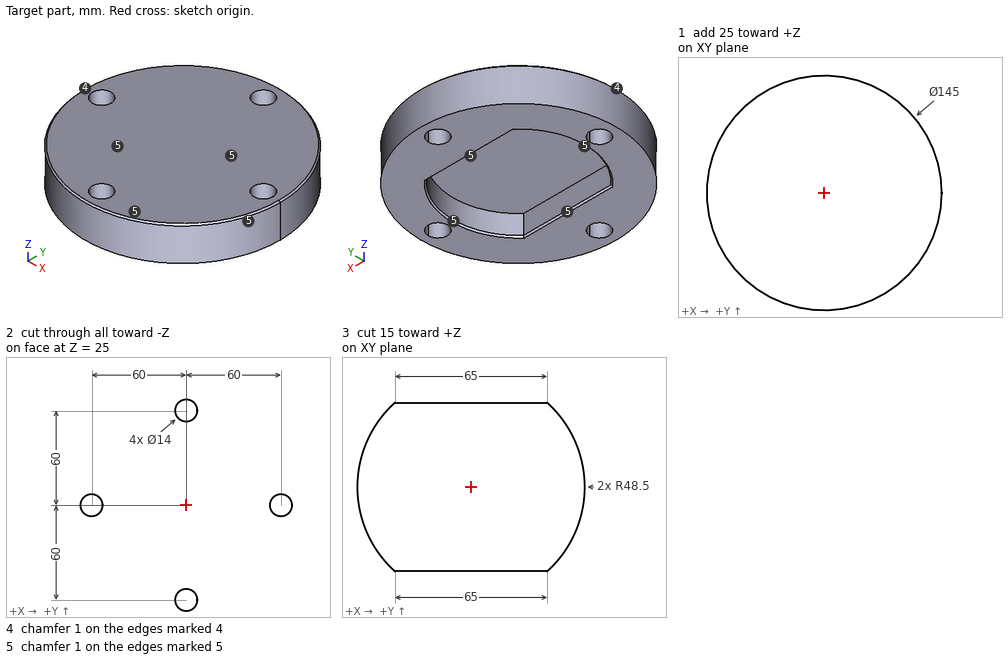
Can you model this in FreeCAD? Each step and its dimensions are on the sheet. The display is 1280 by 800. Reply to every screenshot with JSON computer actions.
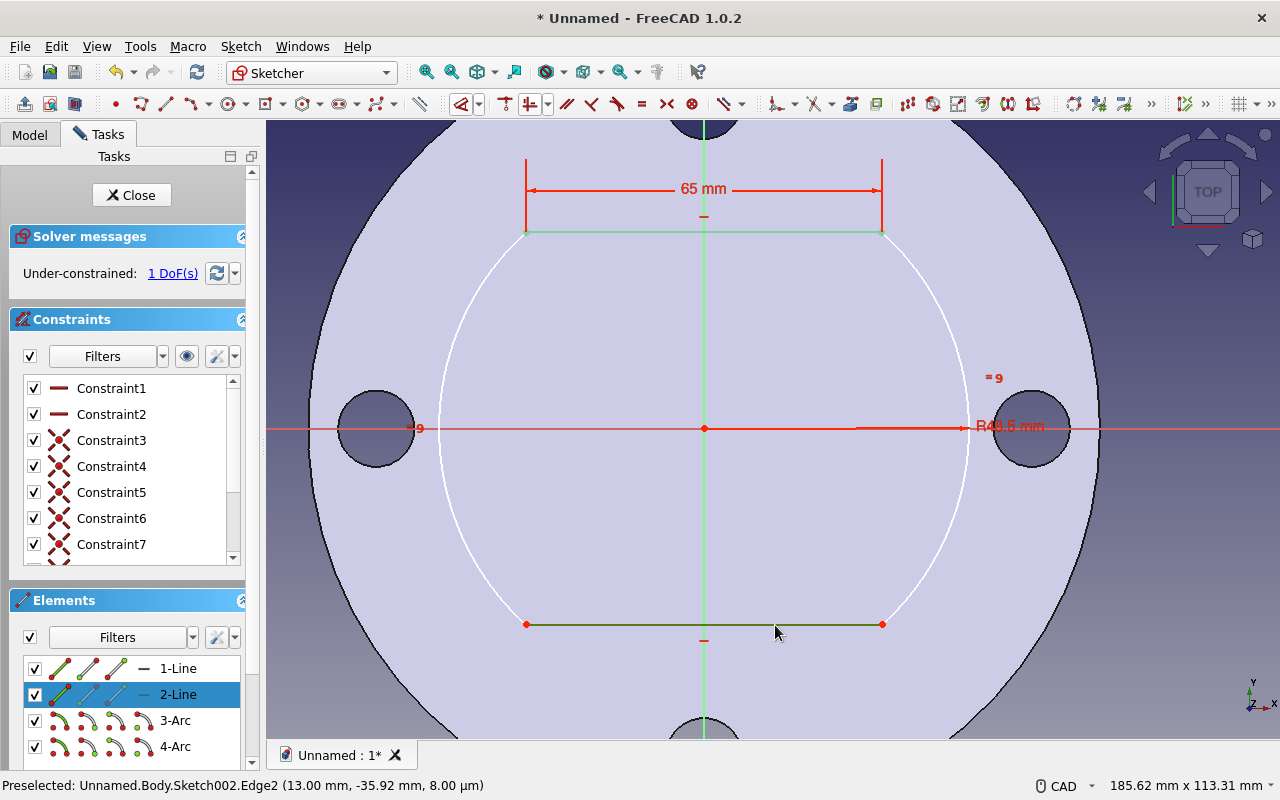
{"action": "left_click", "coordinate": [478, 104]}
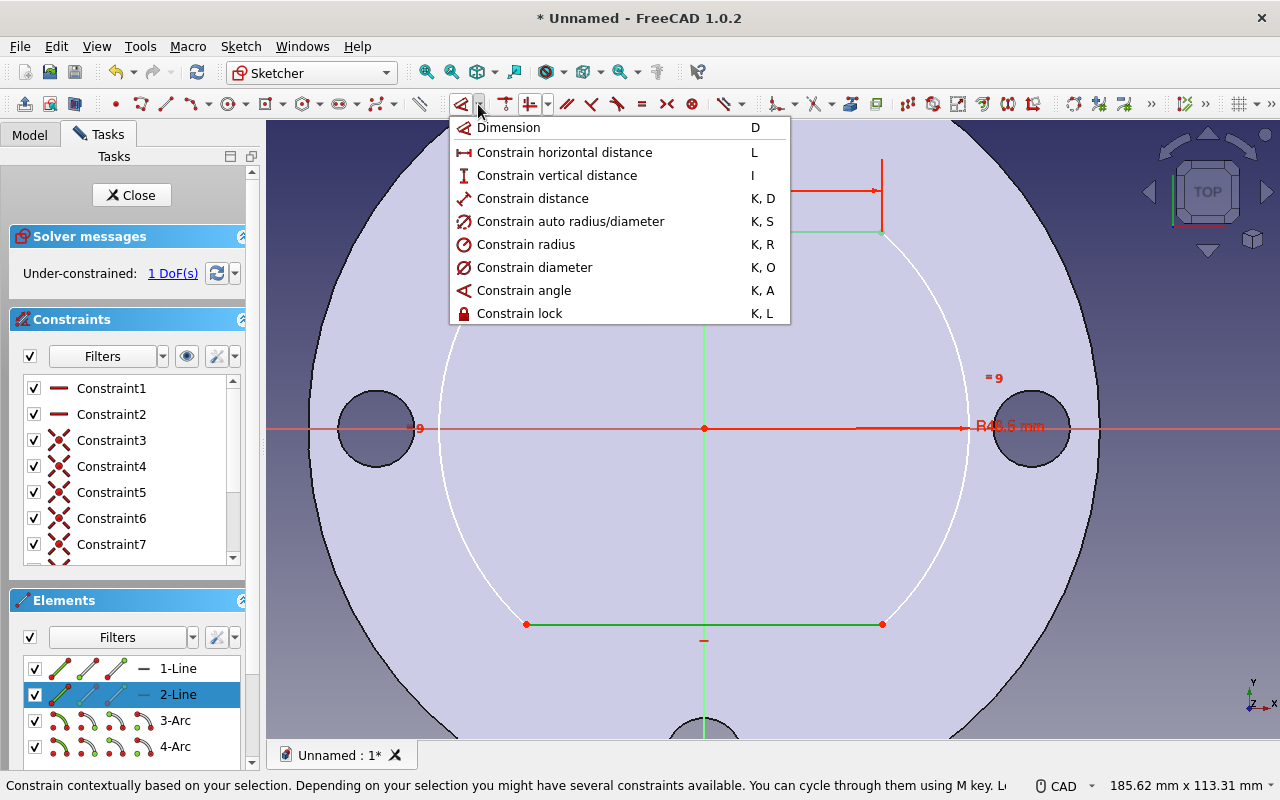
{"action": "left_click", "coordinate": [620, 152]}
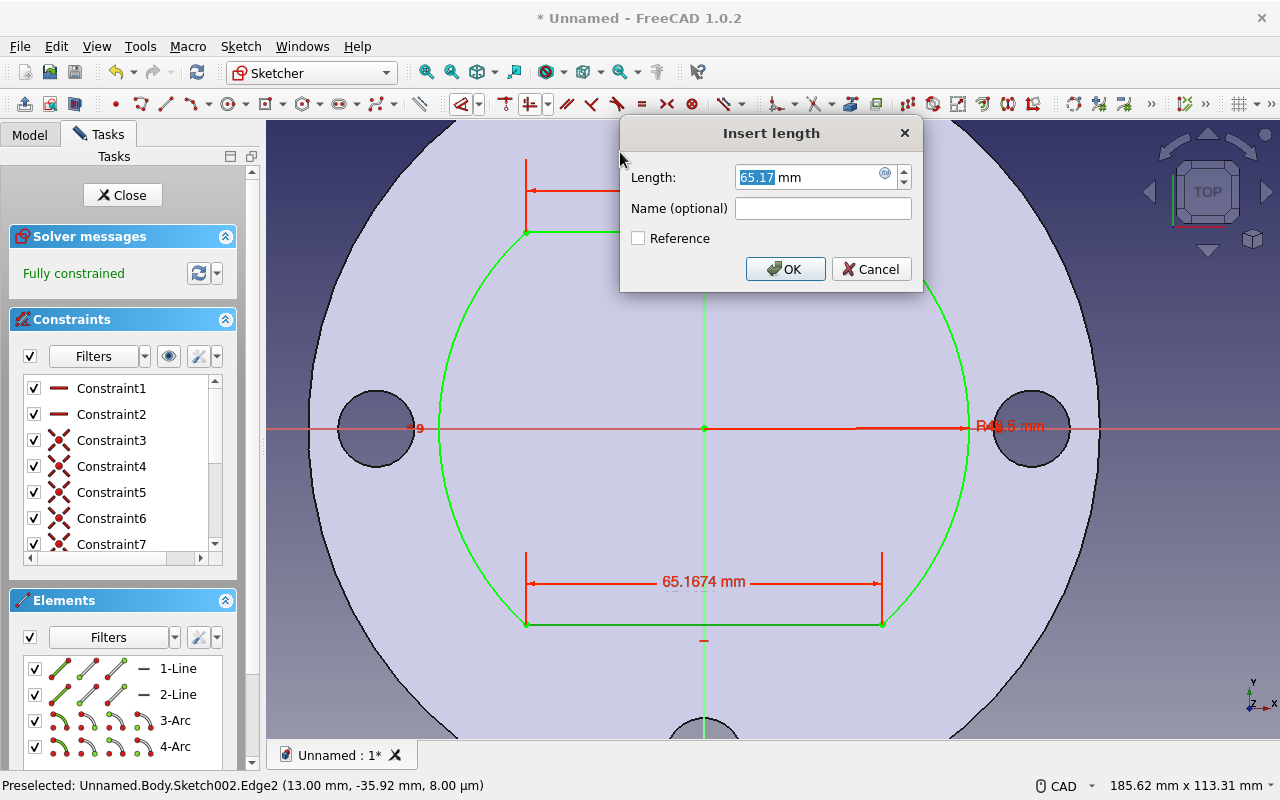
{"action": "type", "text": "65"}
{"action": "key", "text": "Return"}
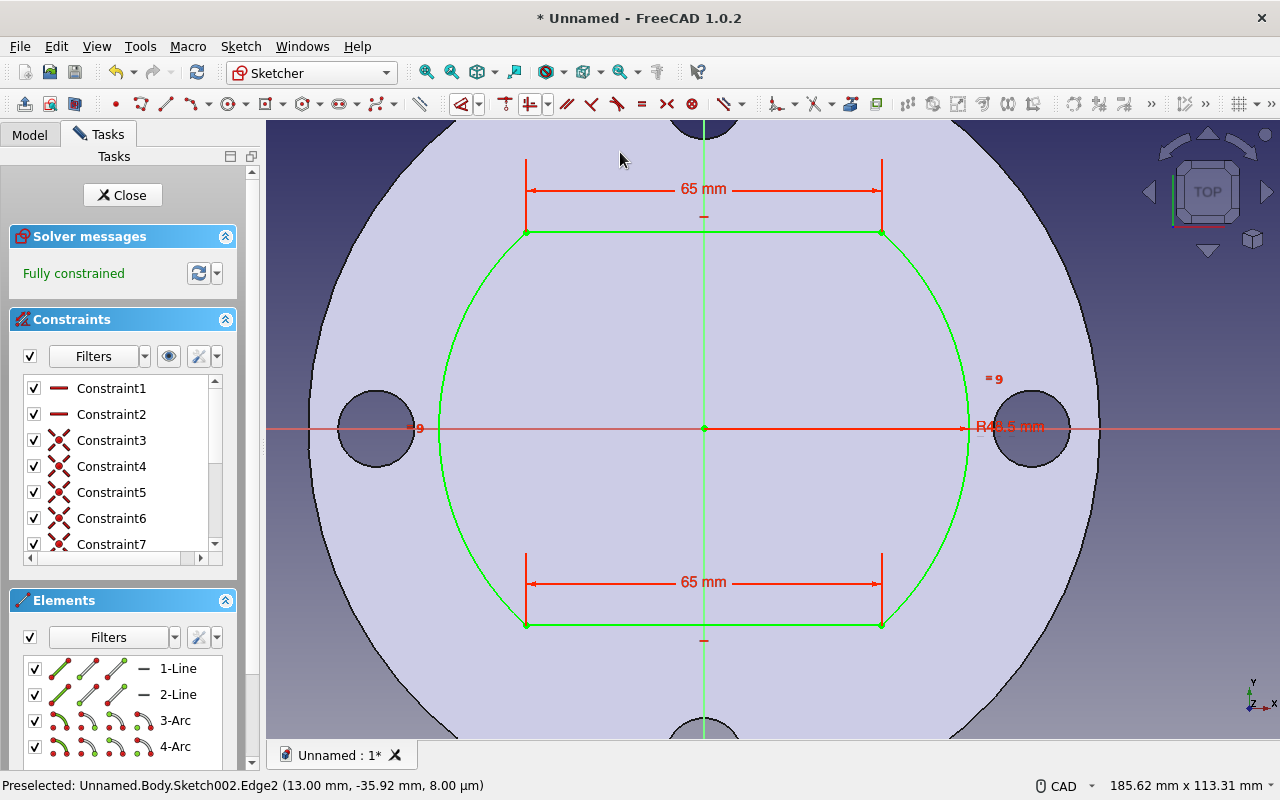
{"action": "left_click", "coordinate": [123, 195]}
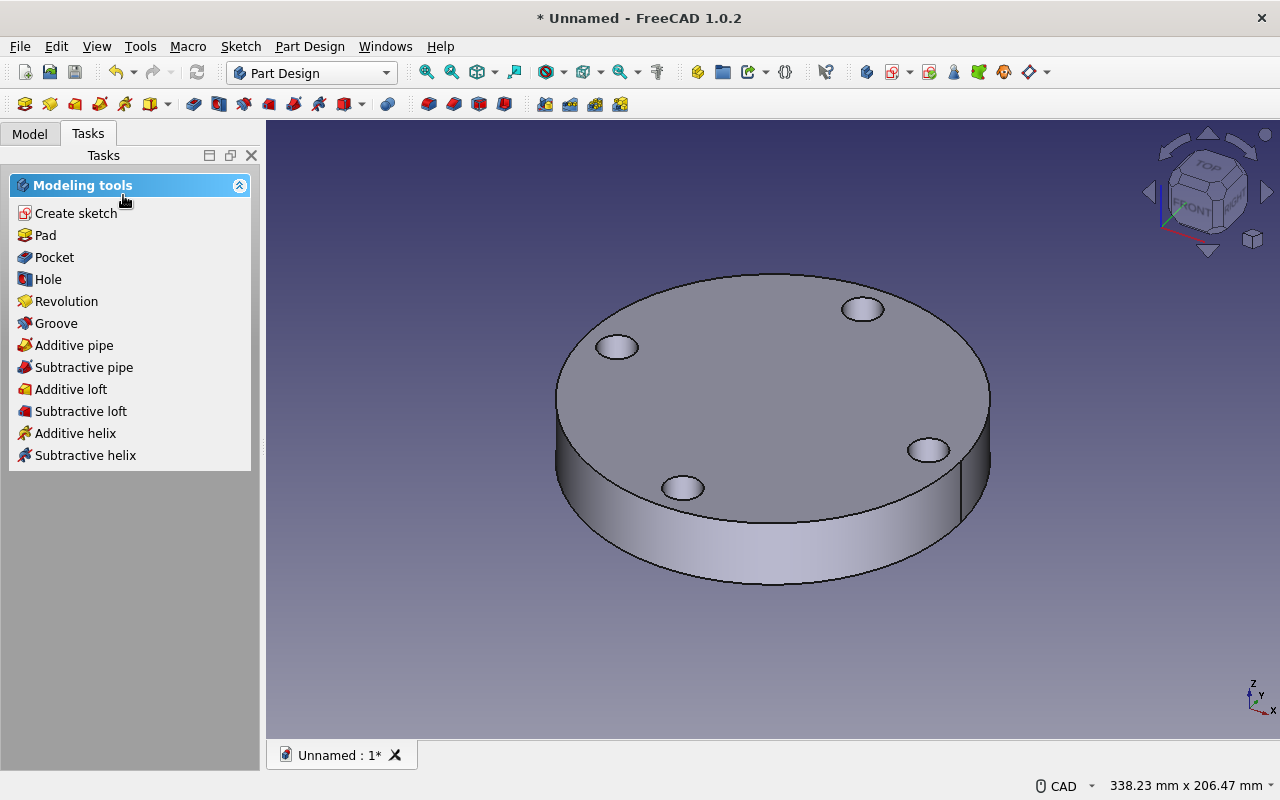
{"action": "left_click", "coordinate": [194, 104]}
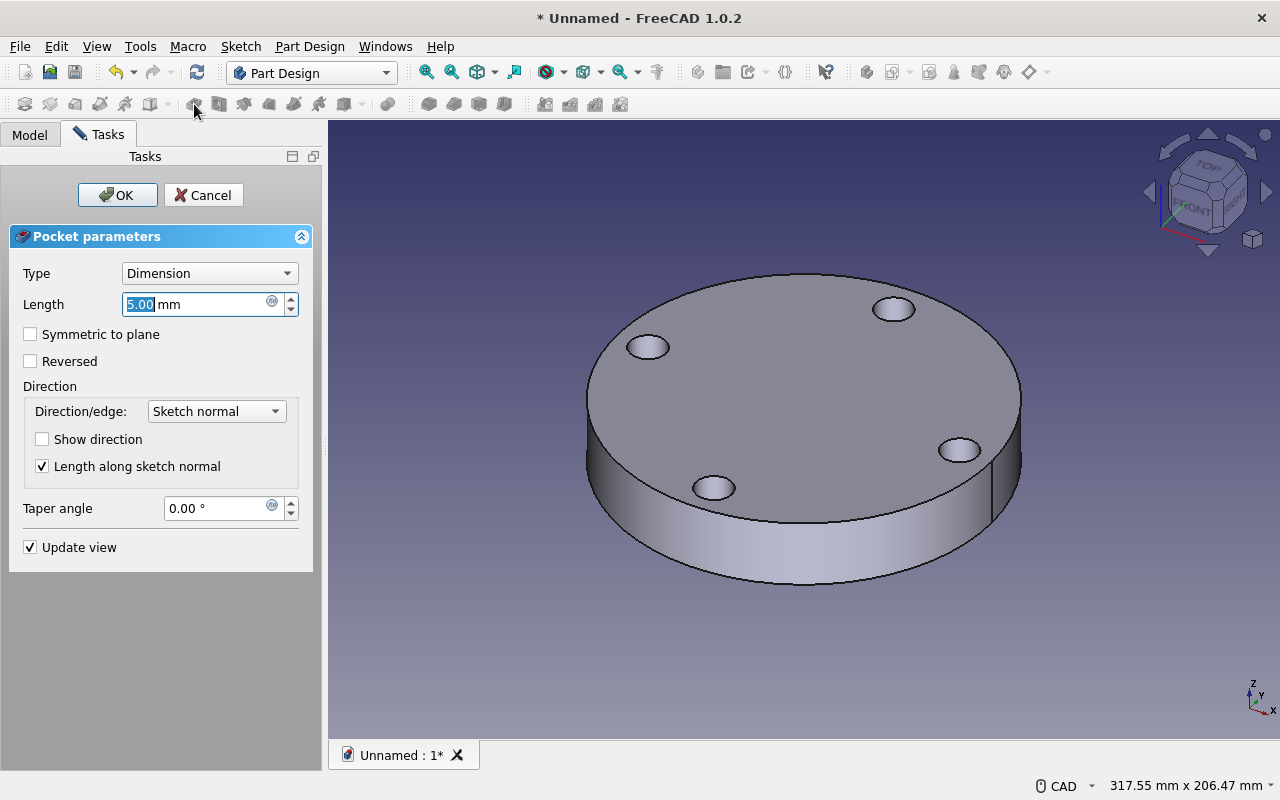
{"action": "type", "text": "15"}
{"action": "key", "text": "Tab"}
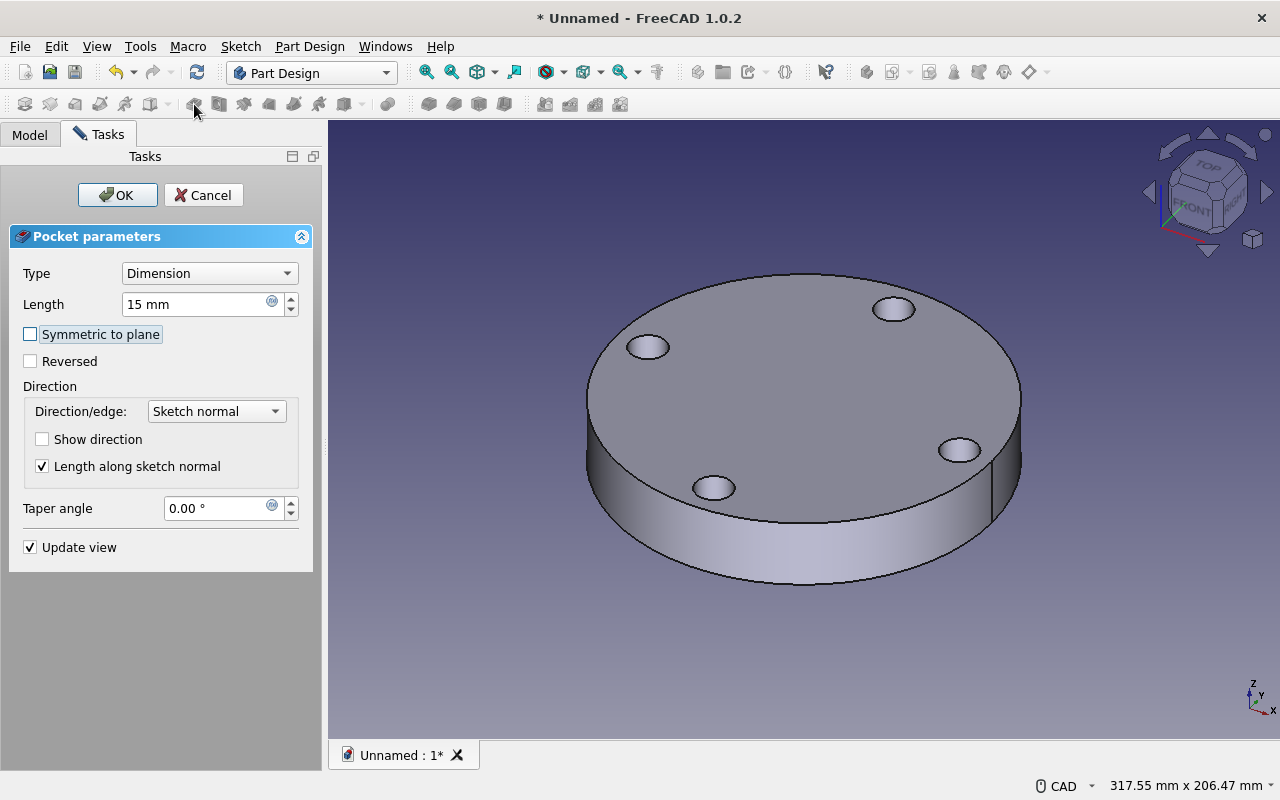
{"action": "left_click", "coordinate": [31, 361]}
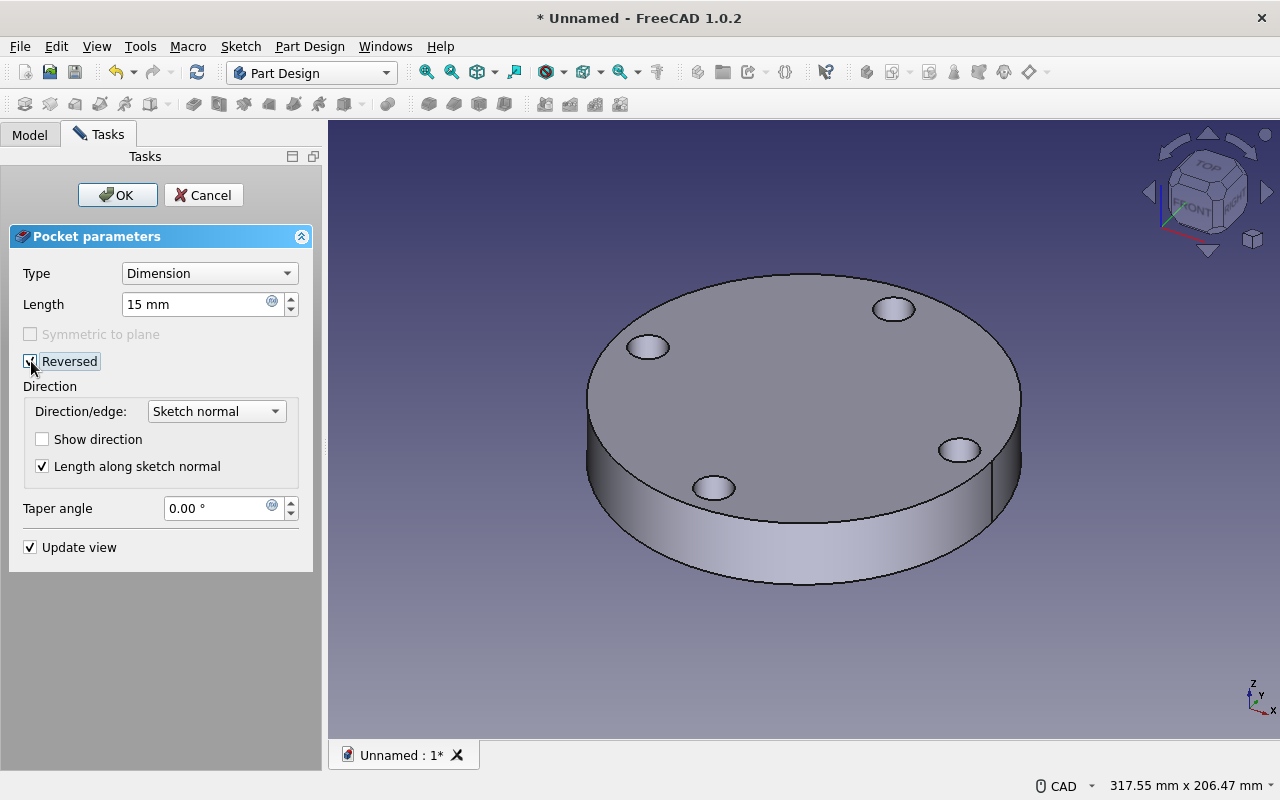
{"action": "left_click", "coordinate": [118, 195]}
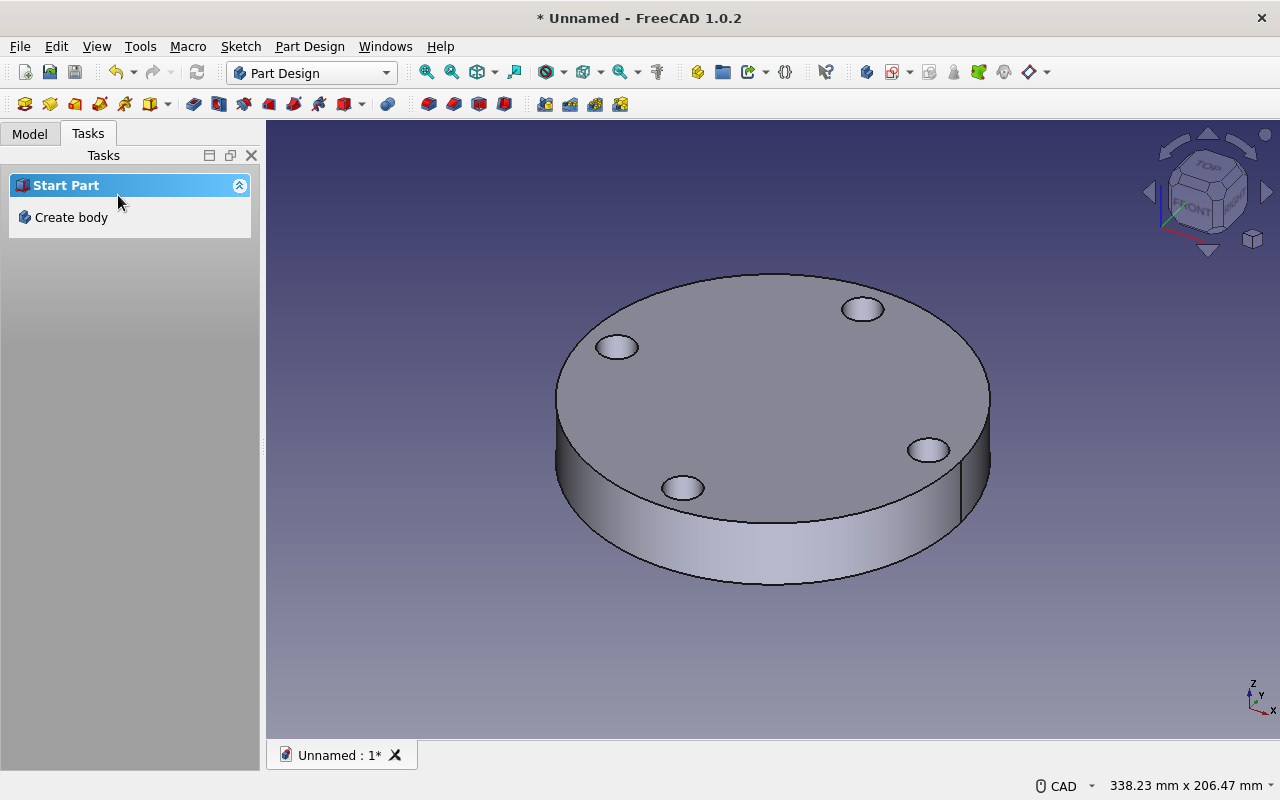
{"action": "left_click", "coordinate": [557, 411]}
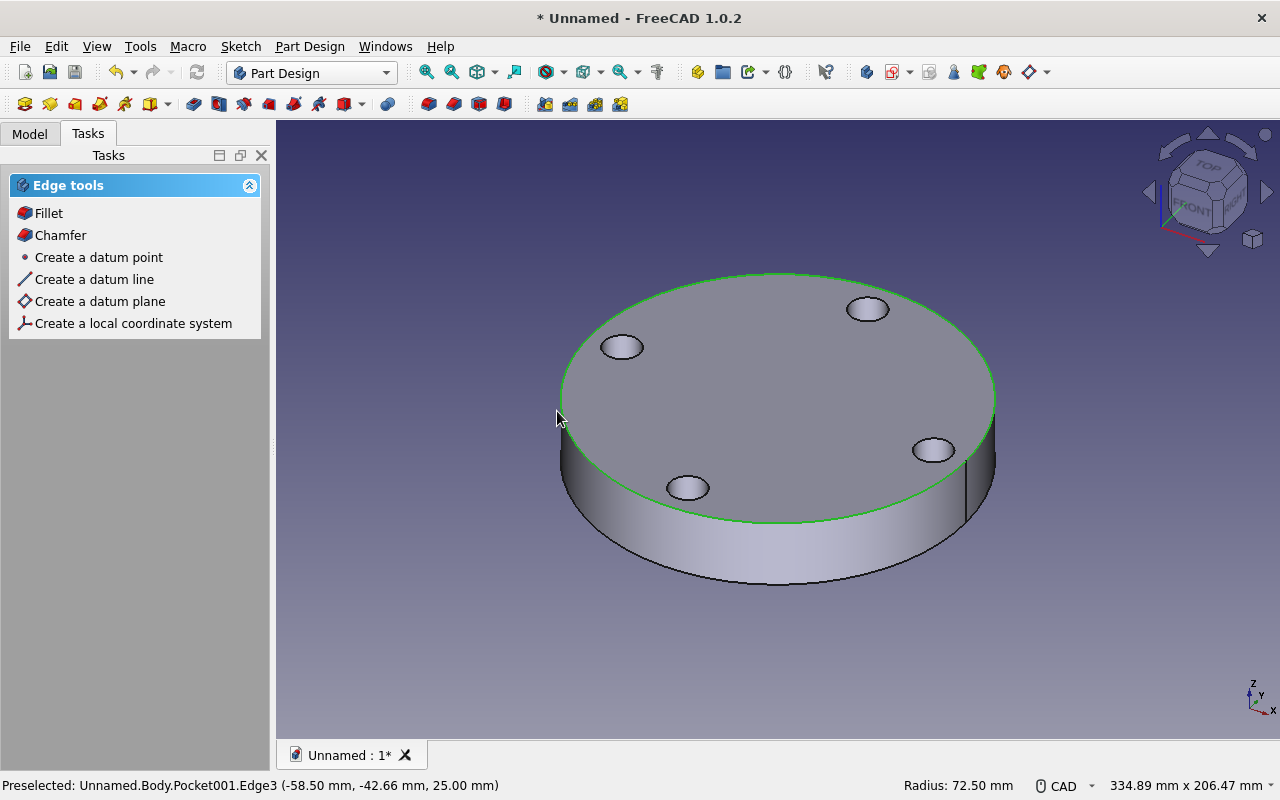
{"action": "left_click", "coordinate": [454, 104]}